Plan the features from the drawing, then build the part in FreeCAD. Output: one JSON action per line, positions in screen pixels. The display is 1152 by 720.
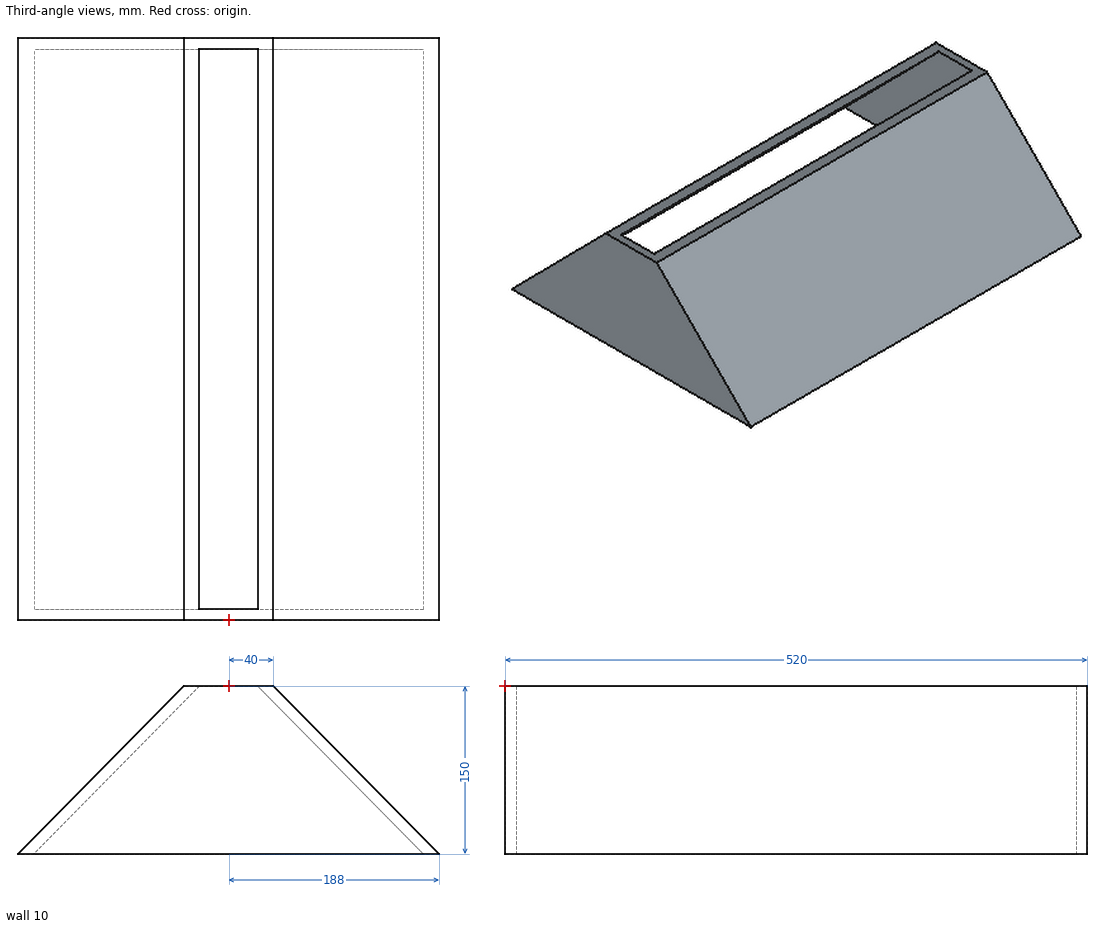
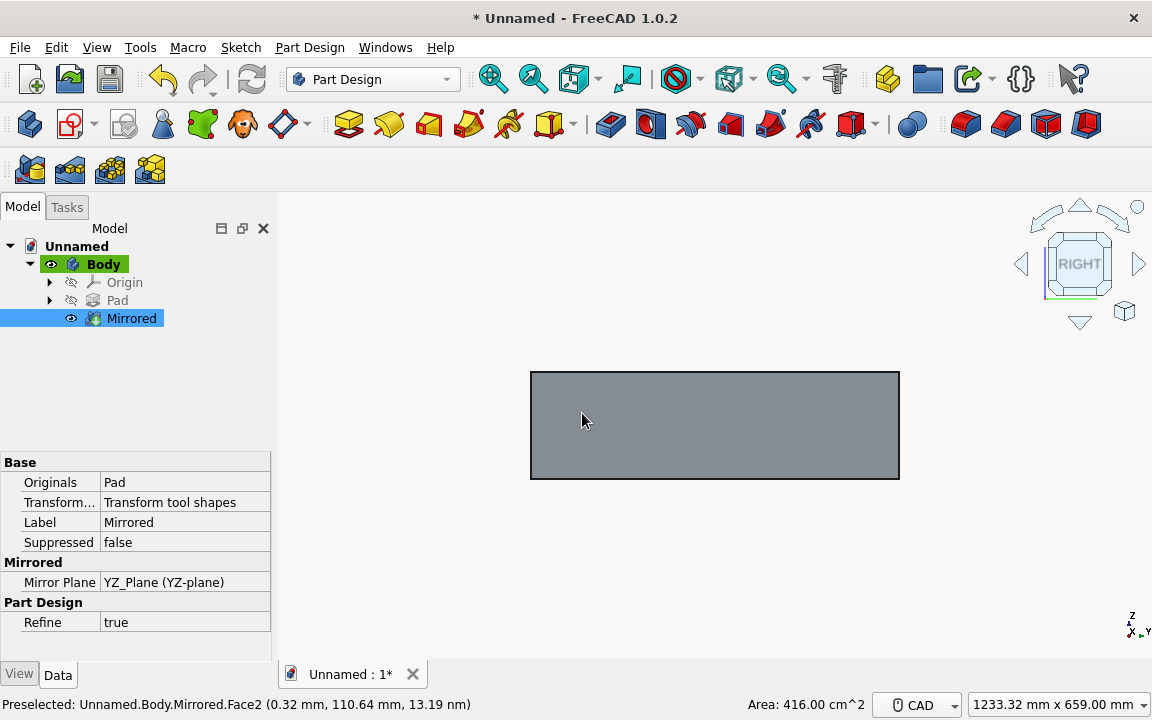
{"action": "key", "text": "v f"}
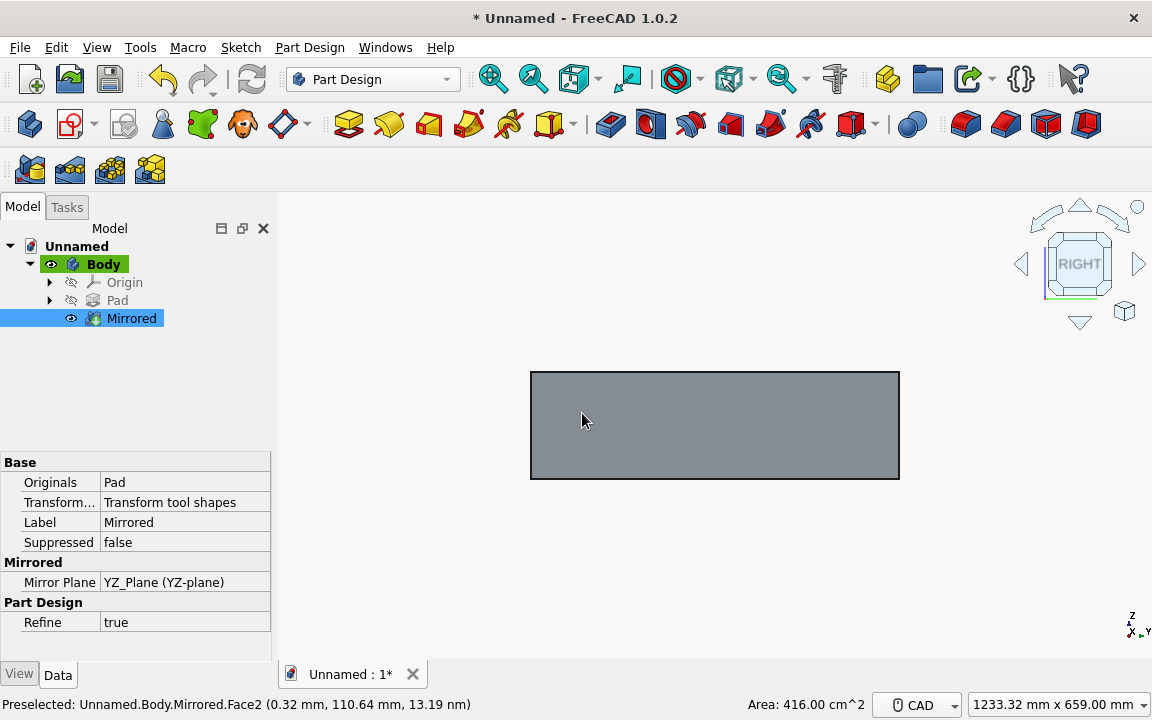
{"action": "key", "text": "5"}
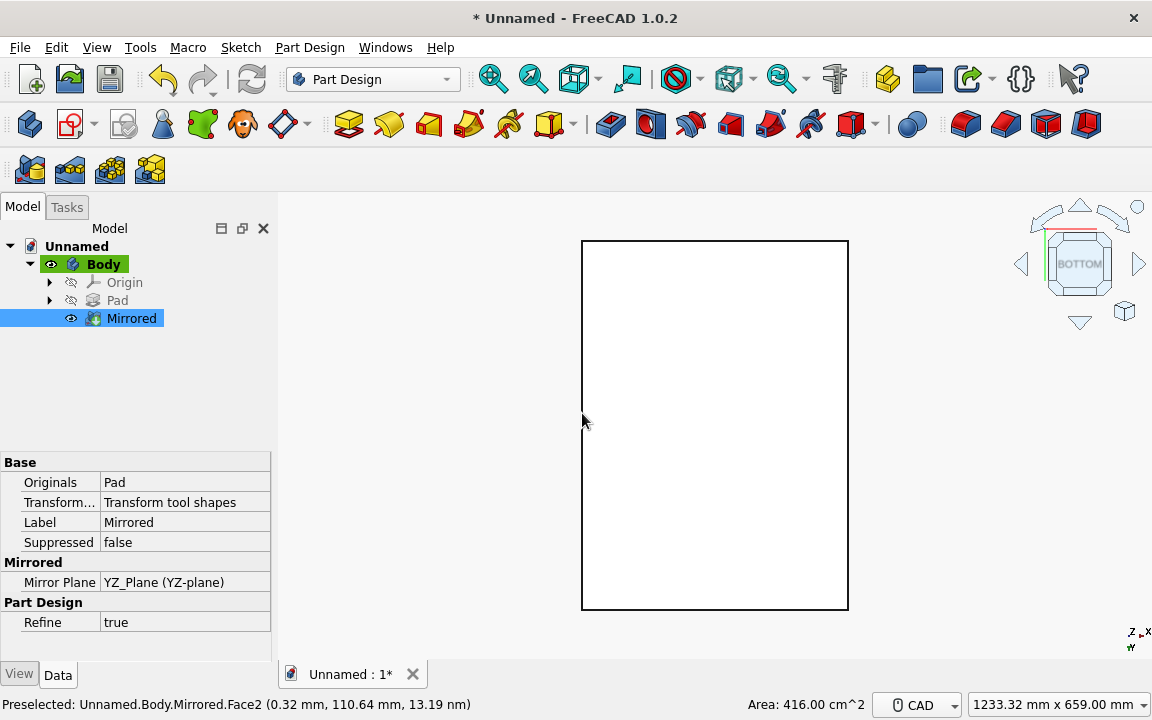
{"action": "left_click", "coordinate": [715, 424], "text": "ctrl"}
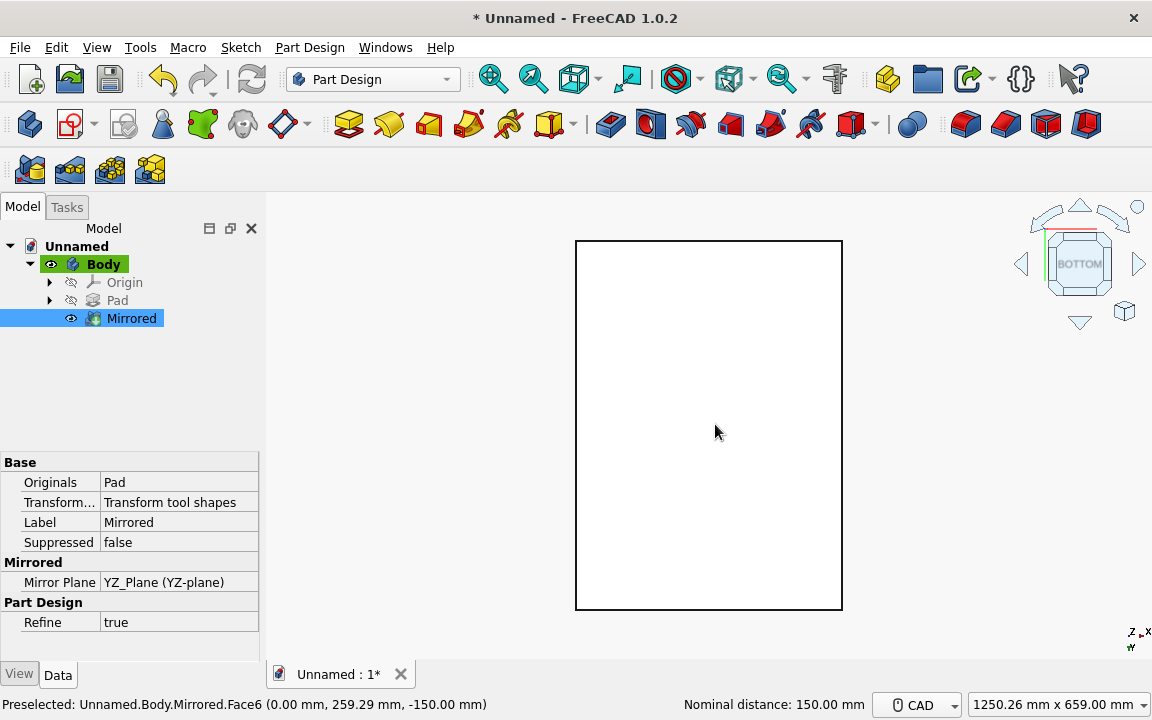
{"action": "left_click", "coordinate": [1086, 124]}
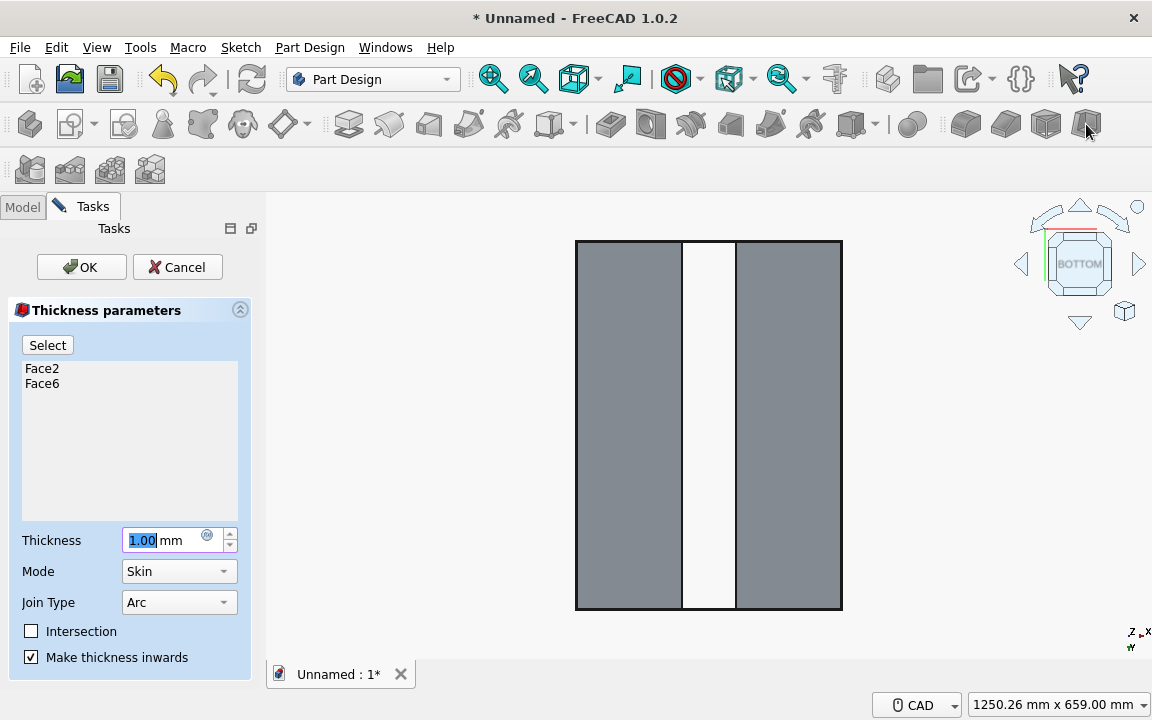
{"action": "type", "text": "10"}
{"action": "key", "text": "Tab"}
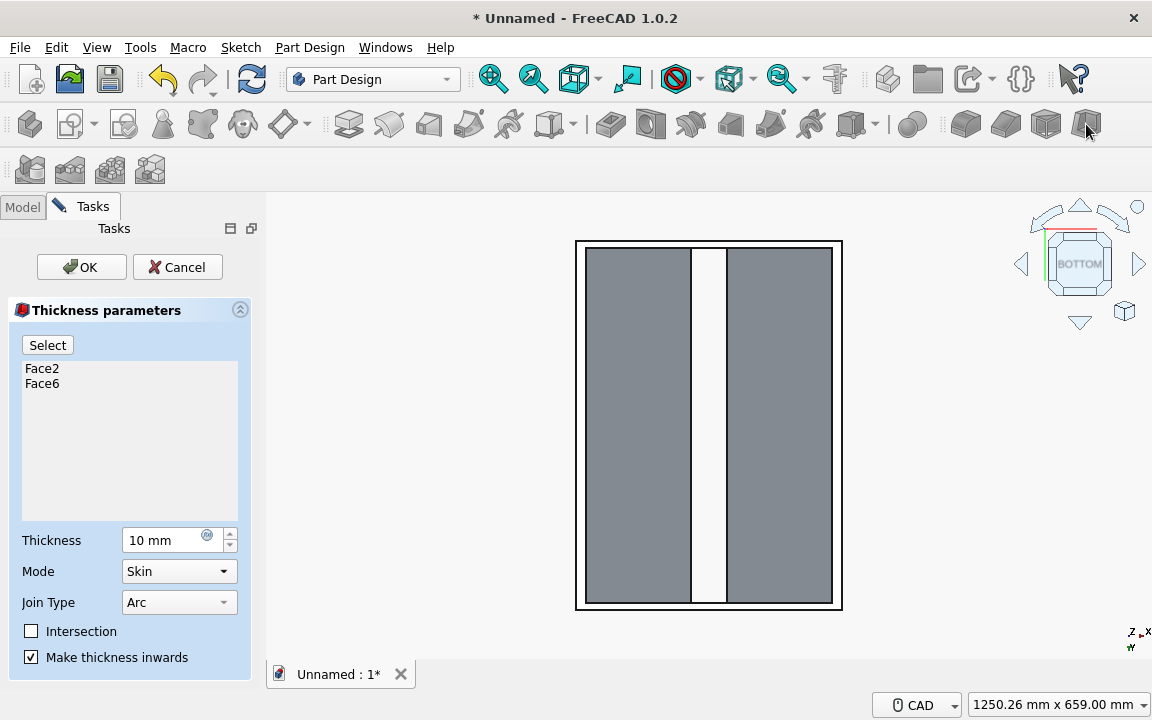
{"action": "left_click", "coordinate": [180, 602]}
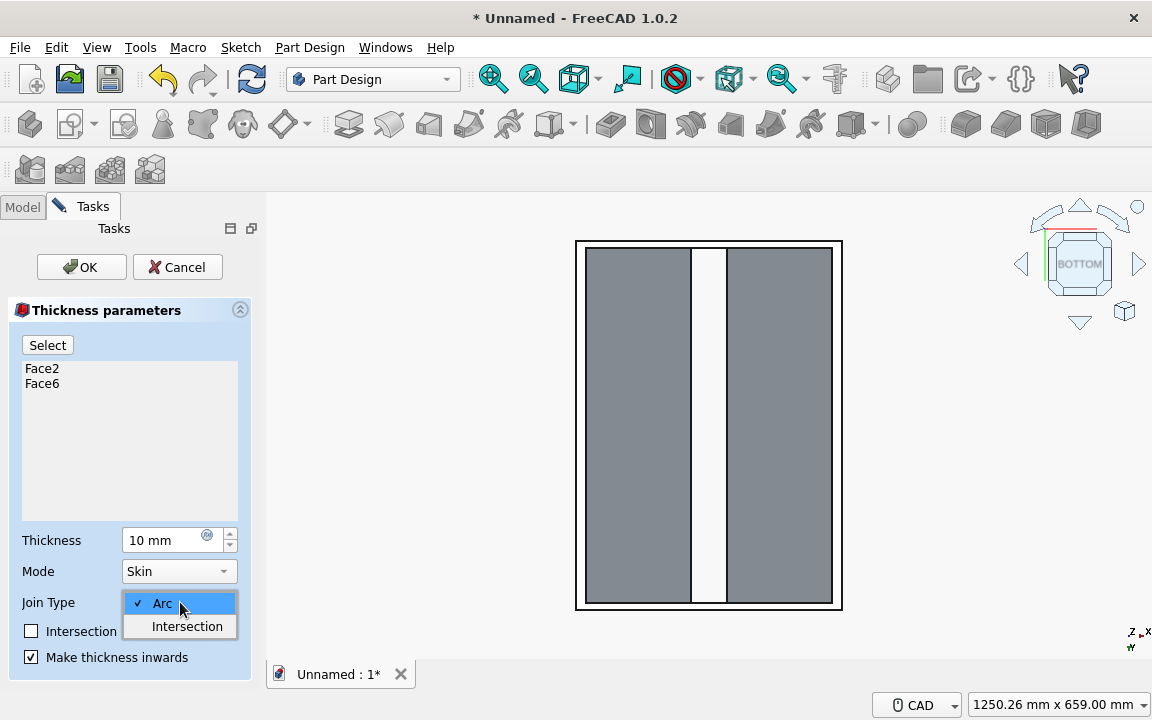
{"action": "left_click", "coordinate": [179, 626]}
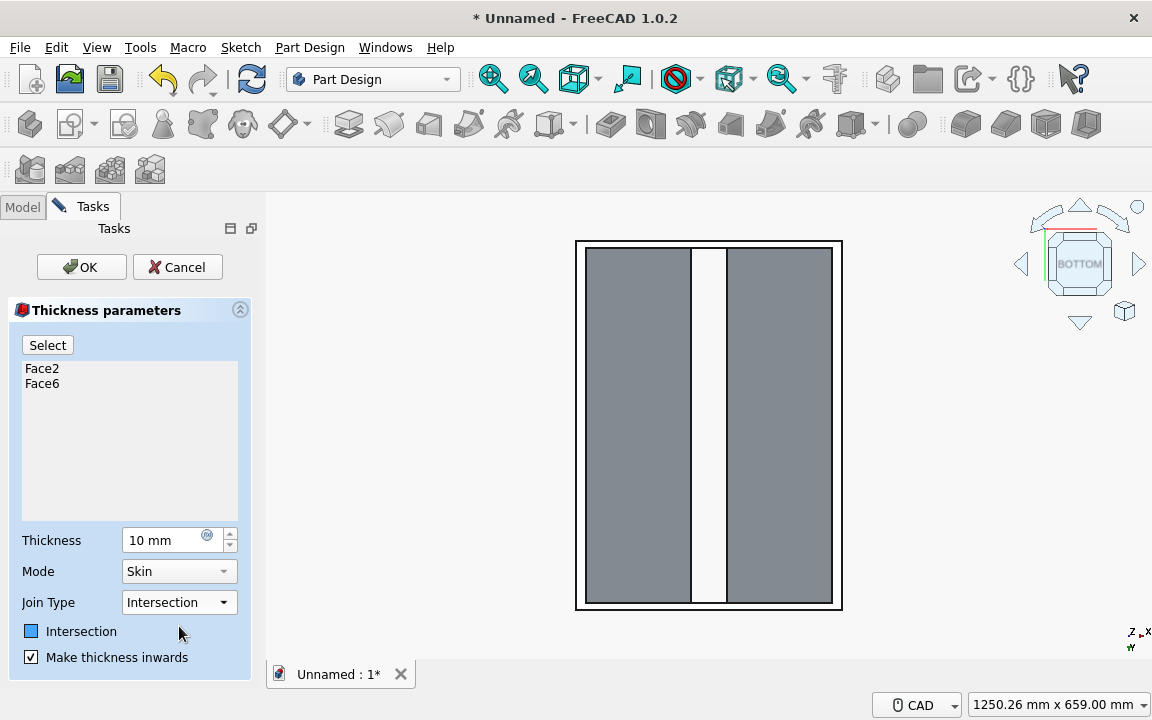
{"action": "left_click", "coordinate": [82, 267]}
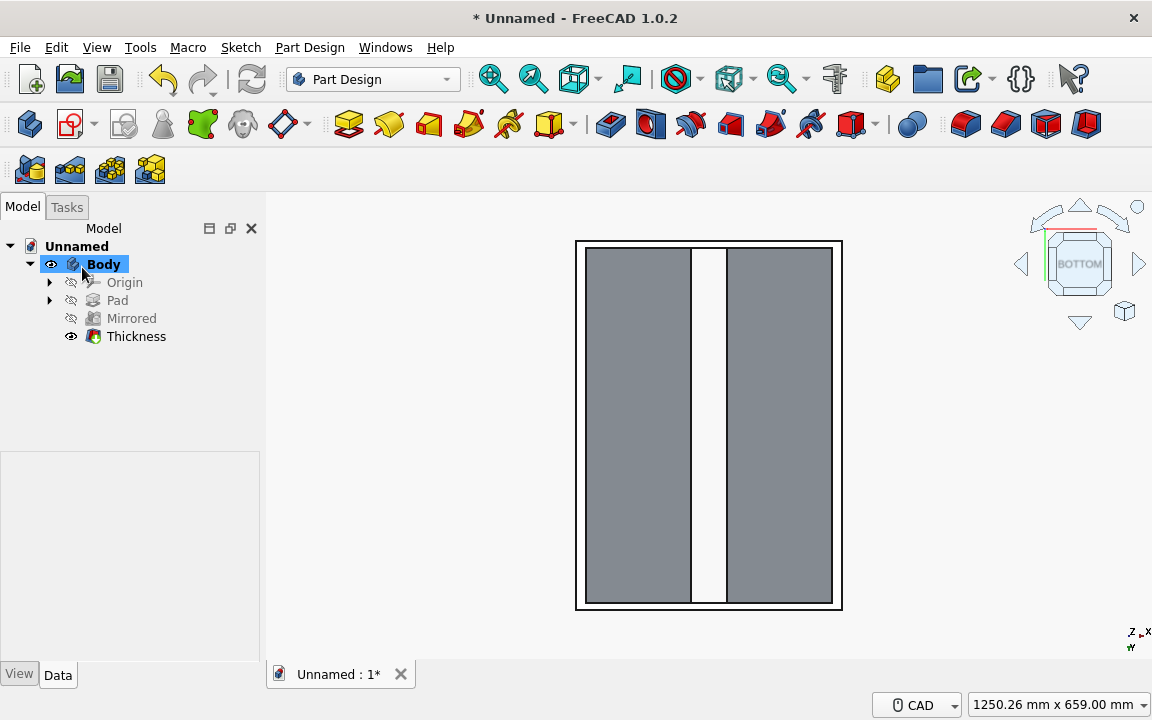
{"action": "key", "text": "0"}